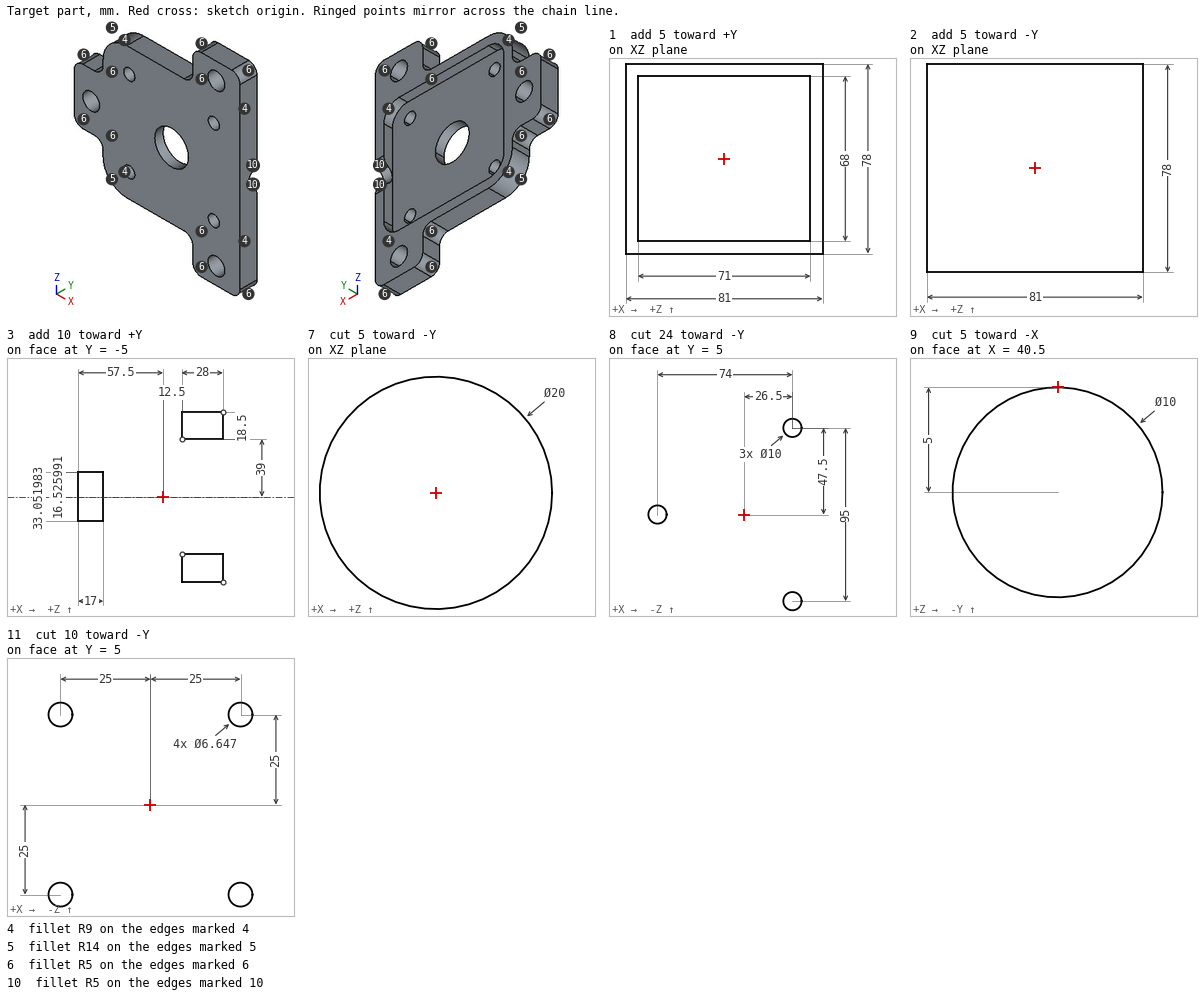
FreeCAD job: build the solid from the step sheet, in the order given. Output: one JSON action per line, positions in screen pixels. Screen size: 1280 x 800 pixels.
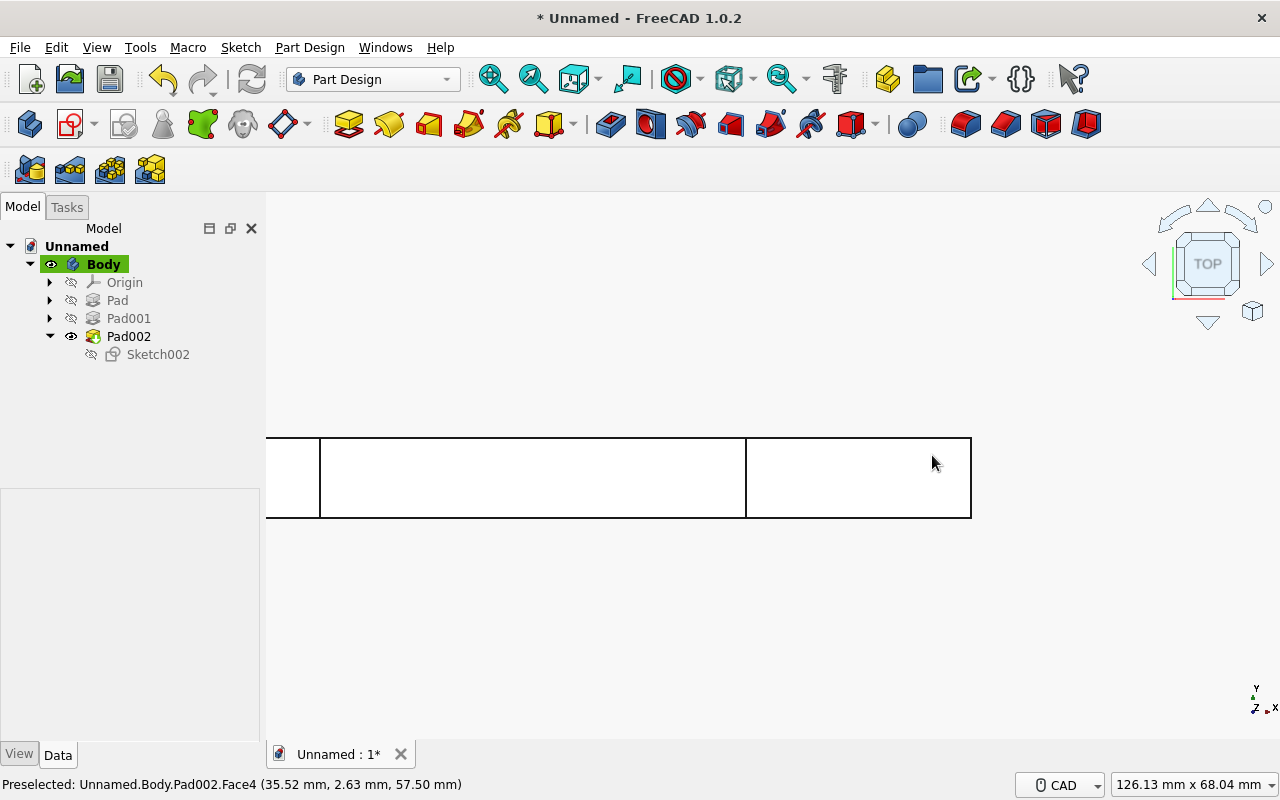
{"action": "key", "text": "v f"}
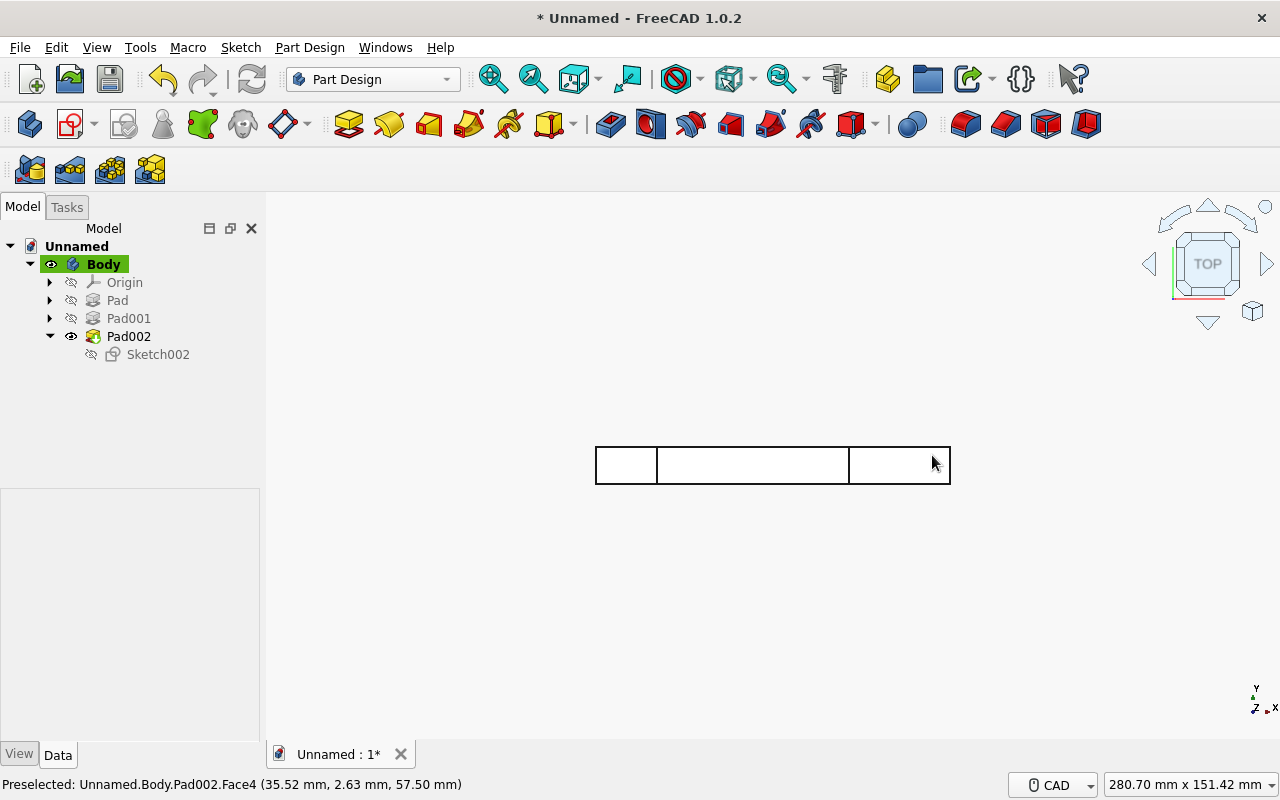
{"action": "key", "text": "1"}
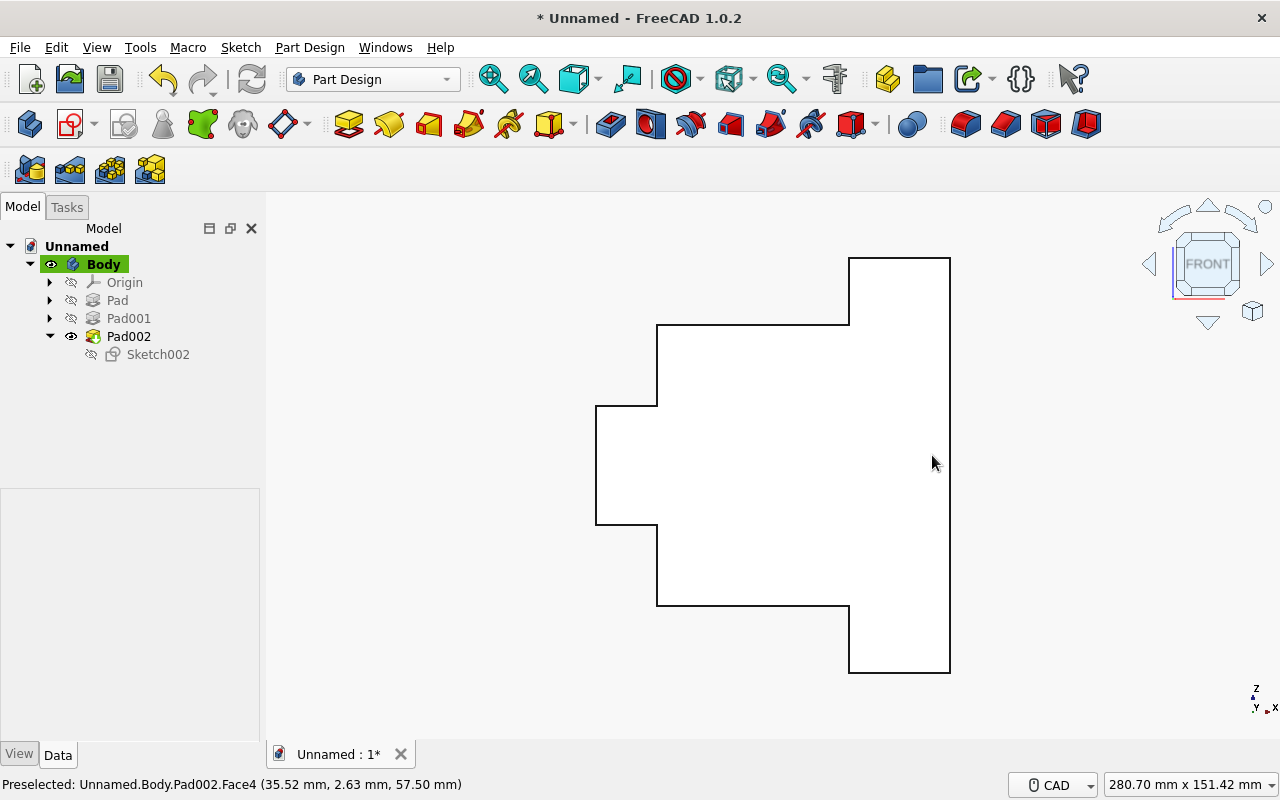
{"action": "scroll", "coordinate": [932, 342], "scroll_direction": "up", "scroll_amount": 4}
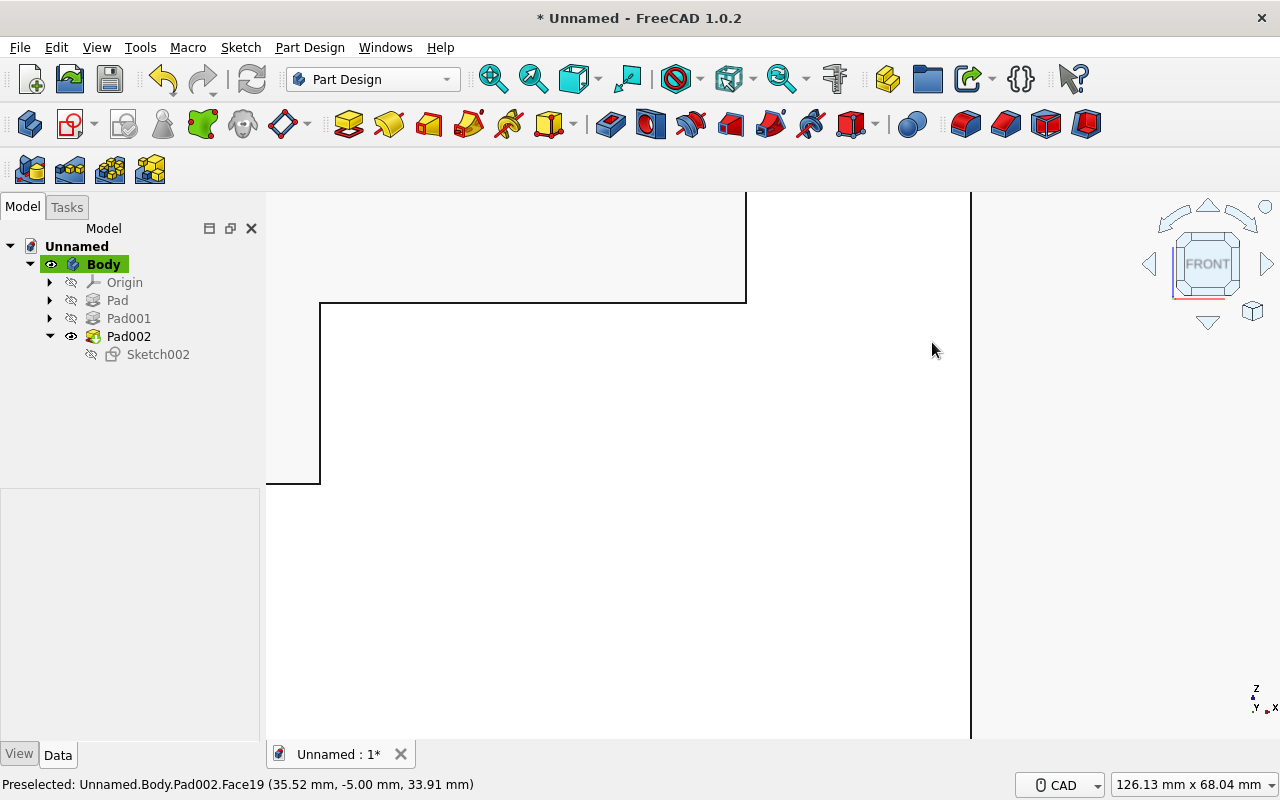
{"action": "key", "text": "v f"}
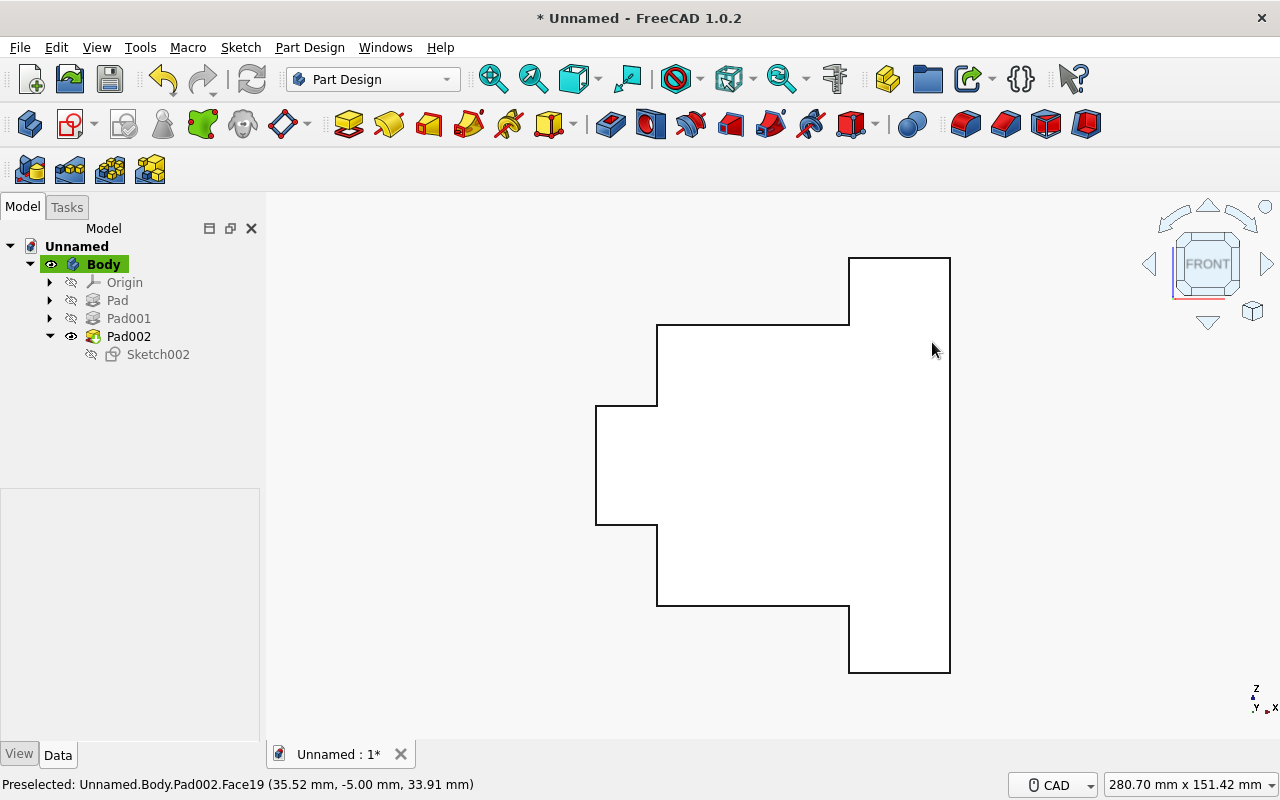
{"action": "key", "text": "3"}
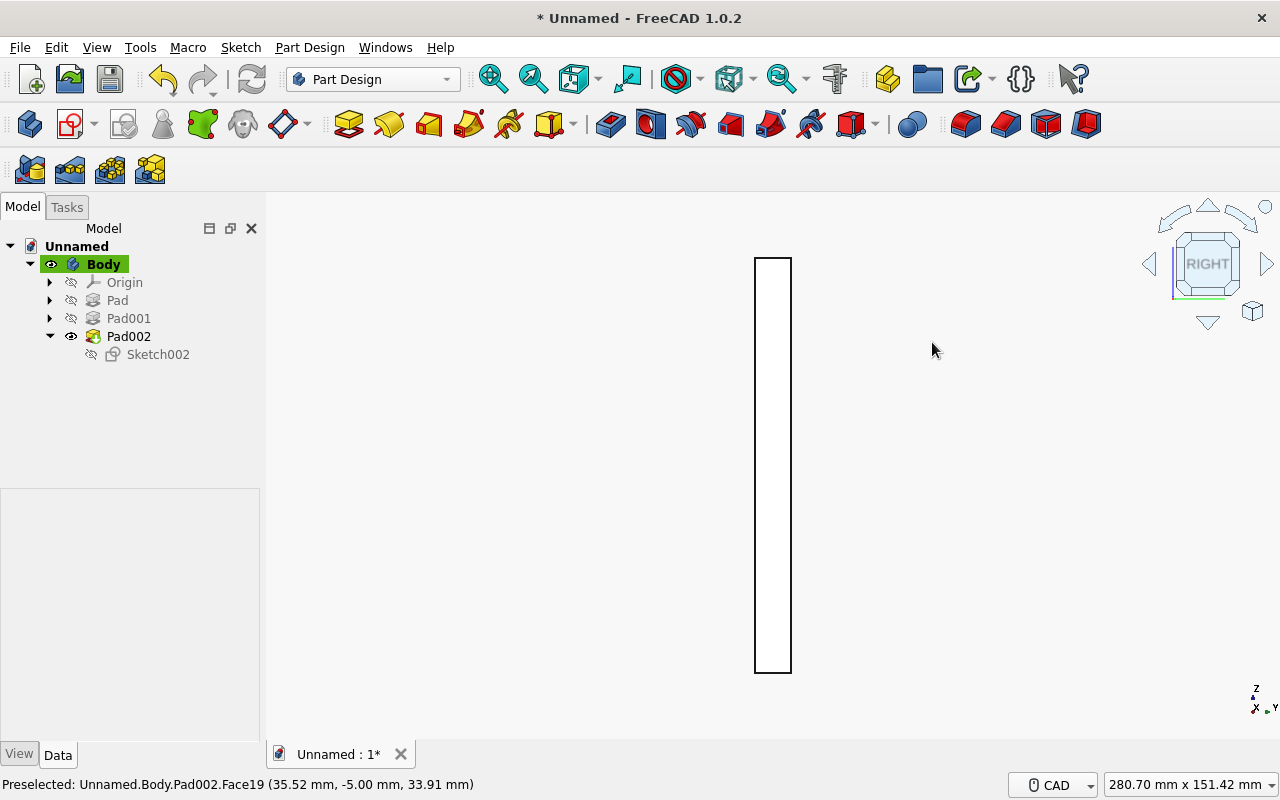
{"action": "scroll", "coordinate": [782, 342], "scroll_direction": "up", "scroll_amount": 4}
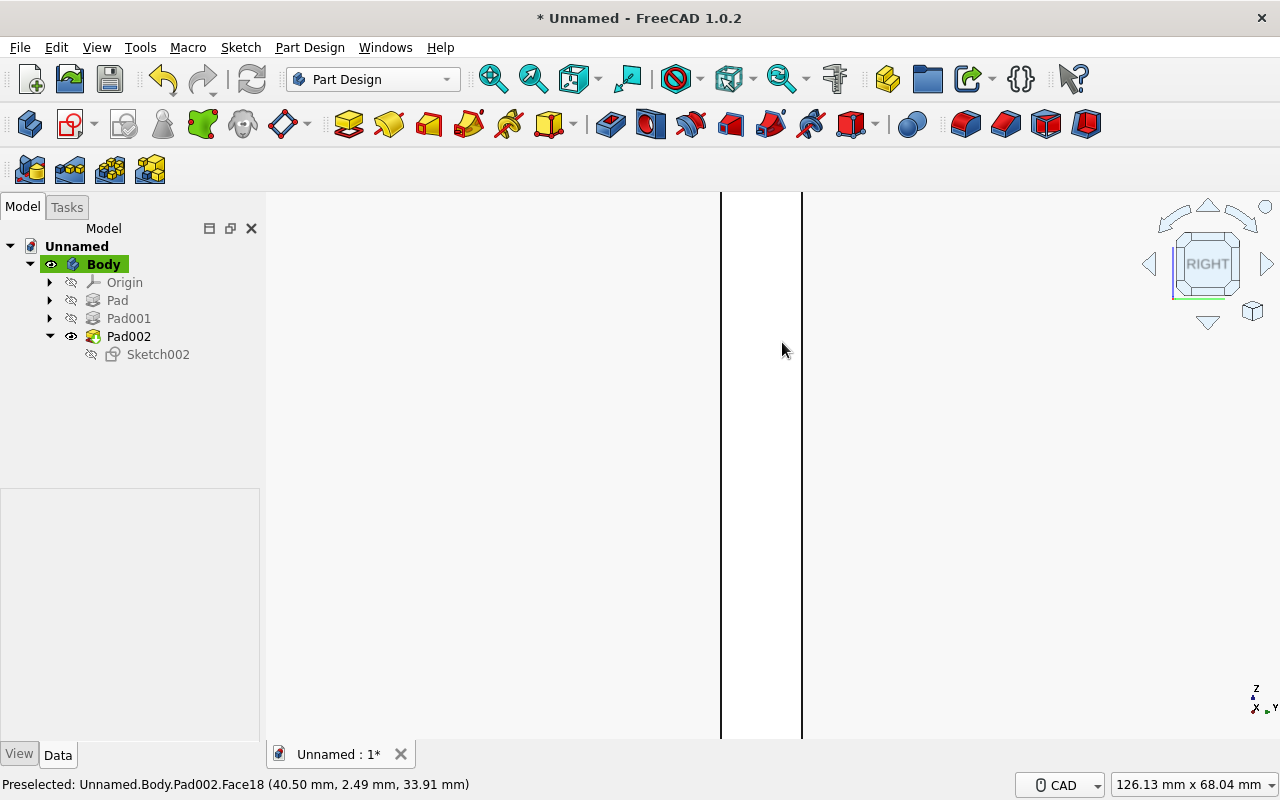
{"action": "left_click", "coordinate": [494, 80]}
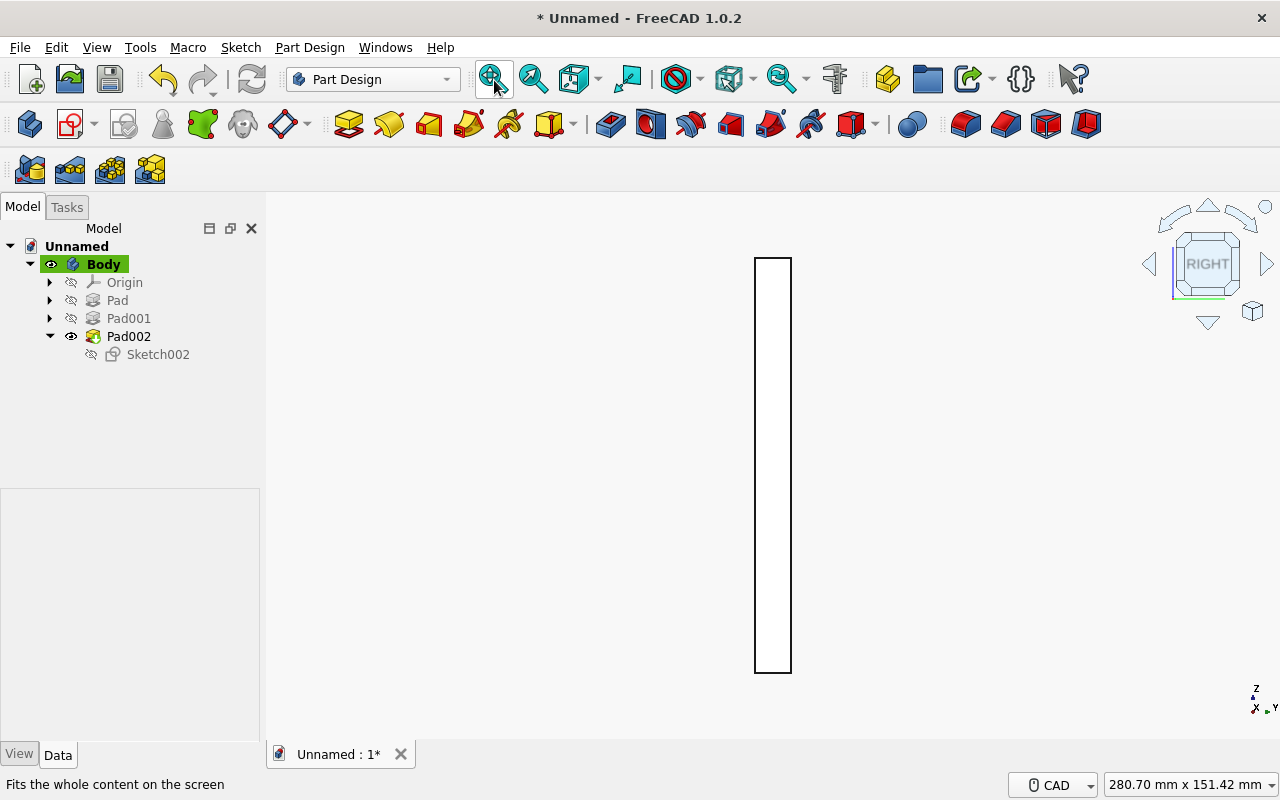
{"action": "key", "text": "5"}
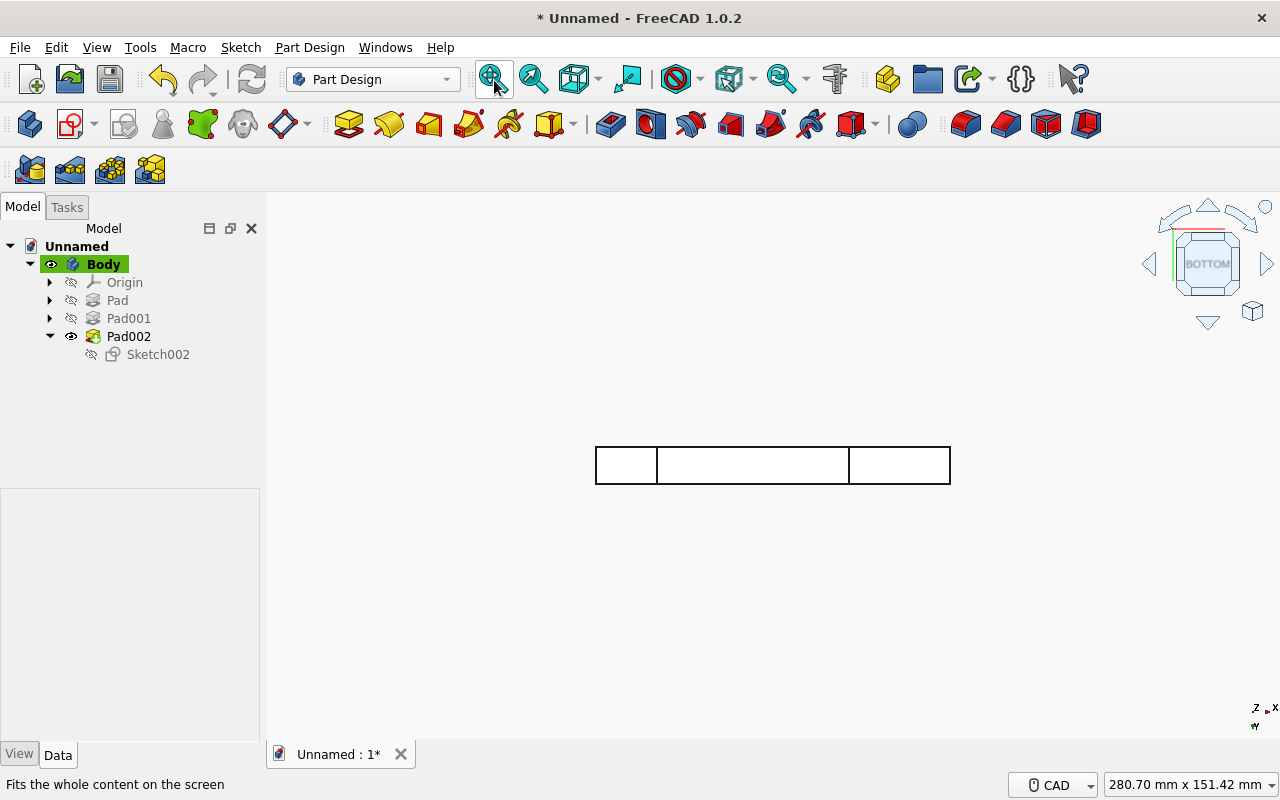
{"action": "key", "text": "v f"}